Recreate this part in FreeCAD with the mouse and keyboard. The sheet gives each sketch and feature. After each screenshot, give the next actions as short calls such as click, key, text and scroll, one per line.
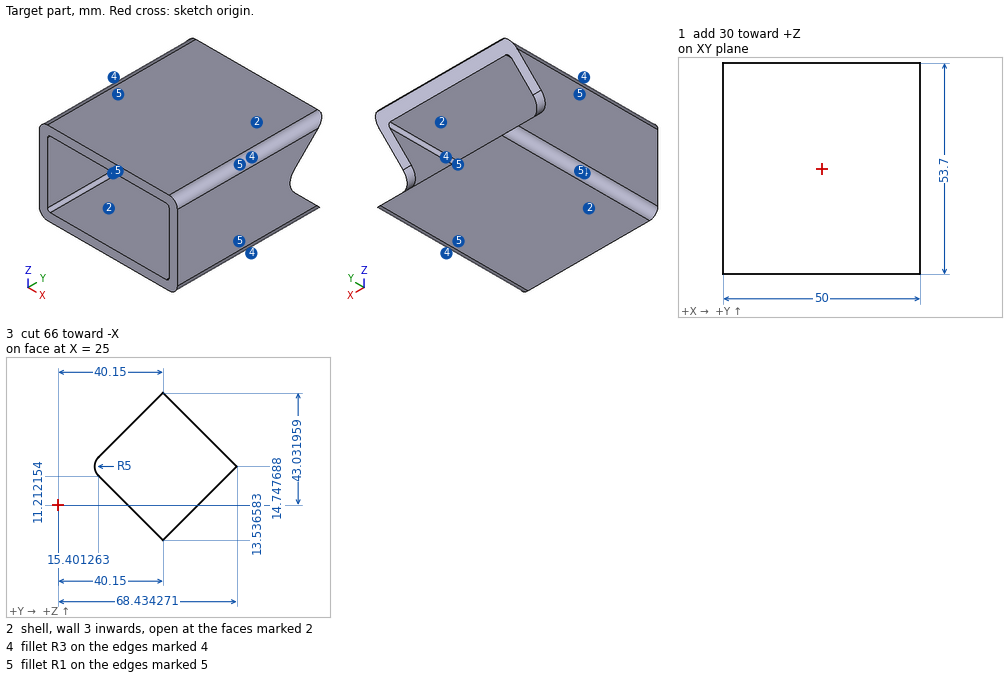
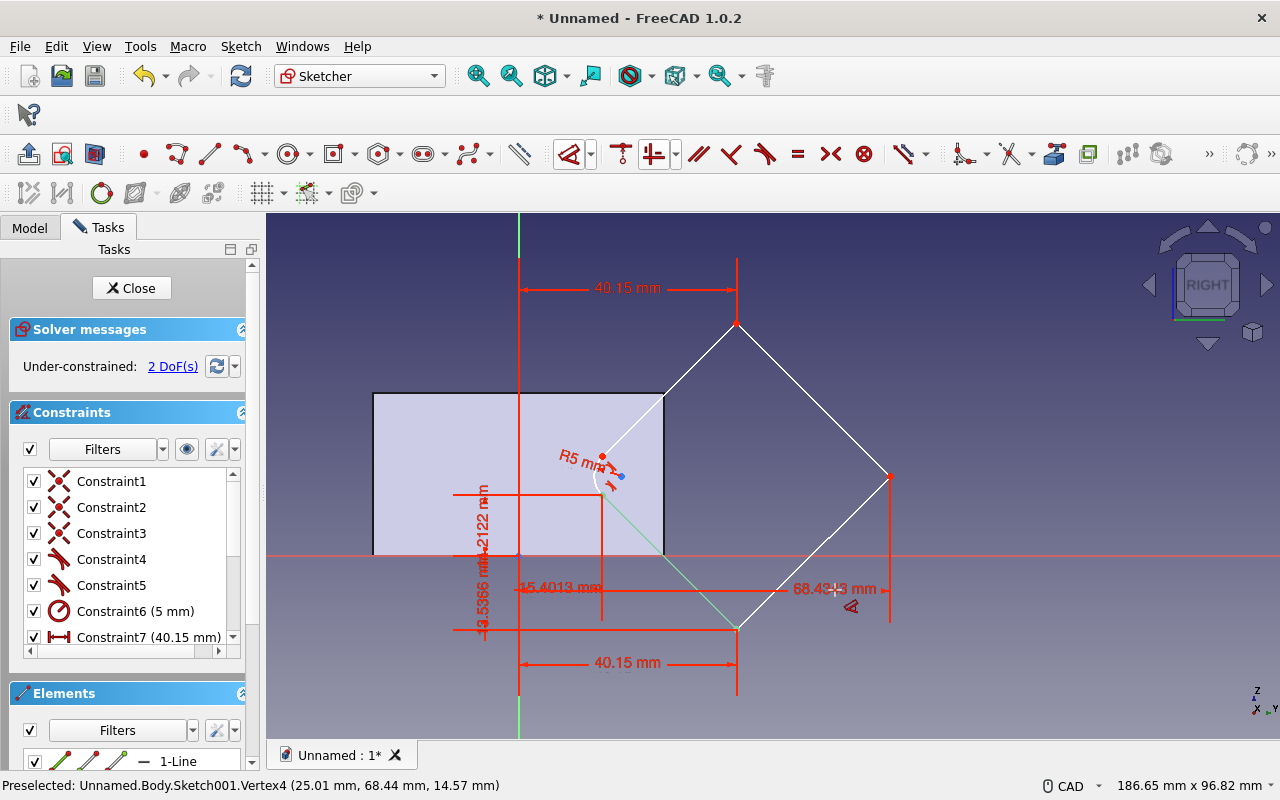
click(890, 477)
click(485, 498)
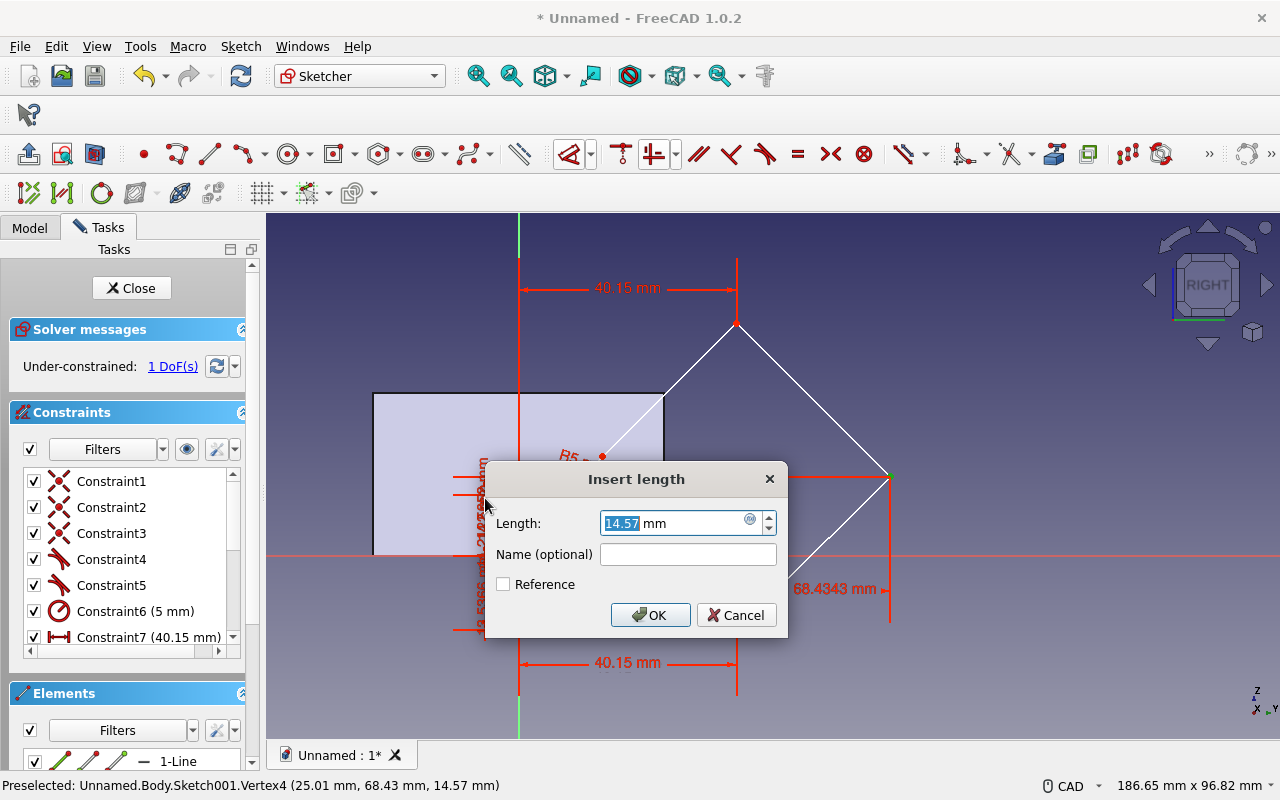
text(14.747688)
key(Return)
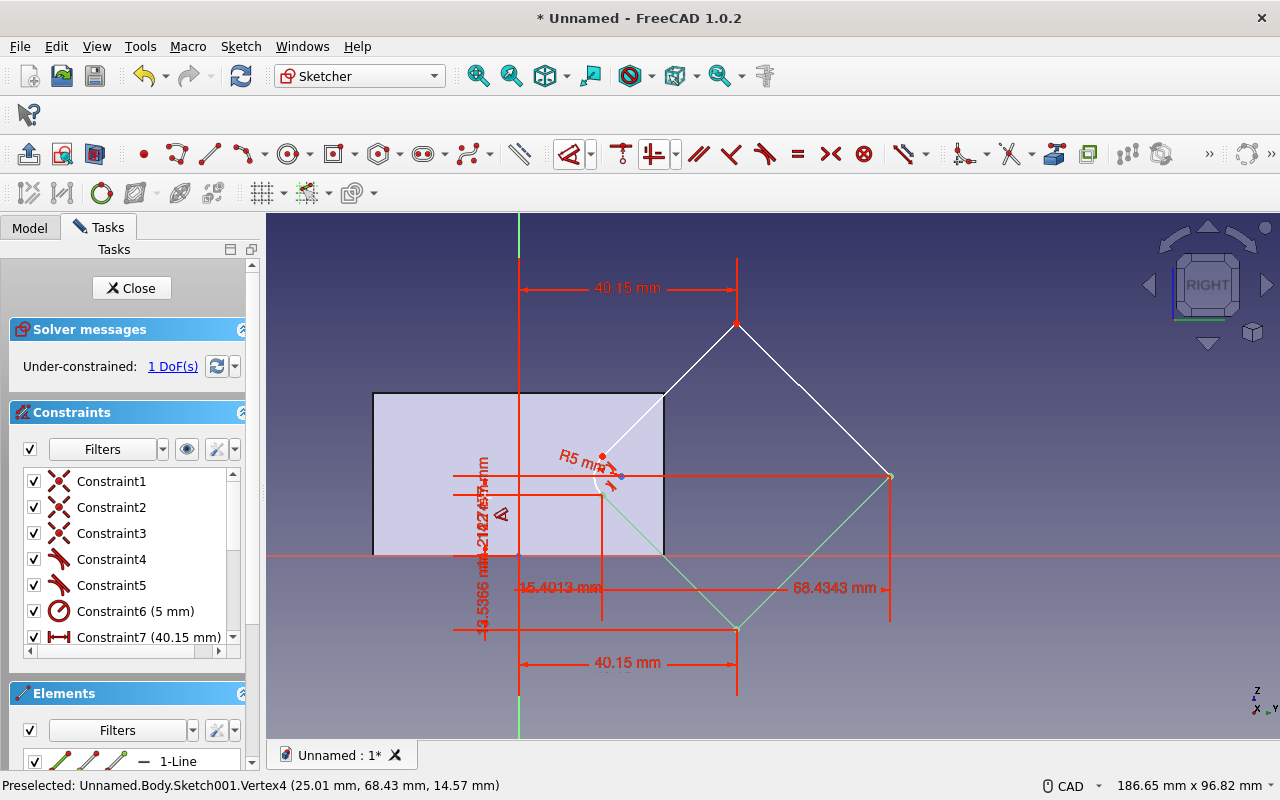
click(737, 323)
click(485, 440)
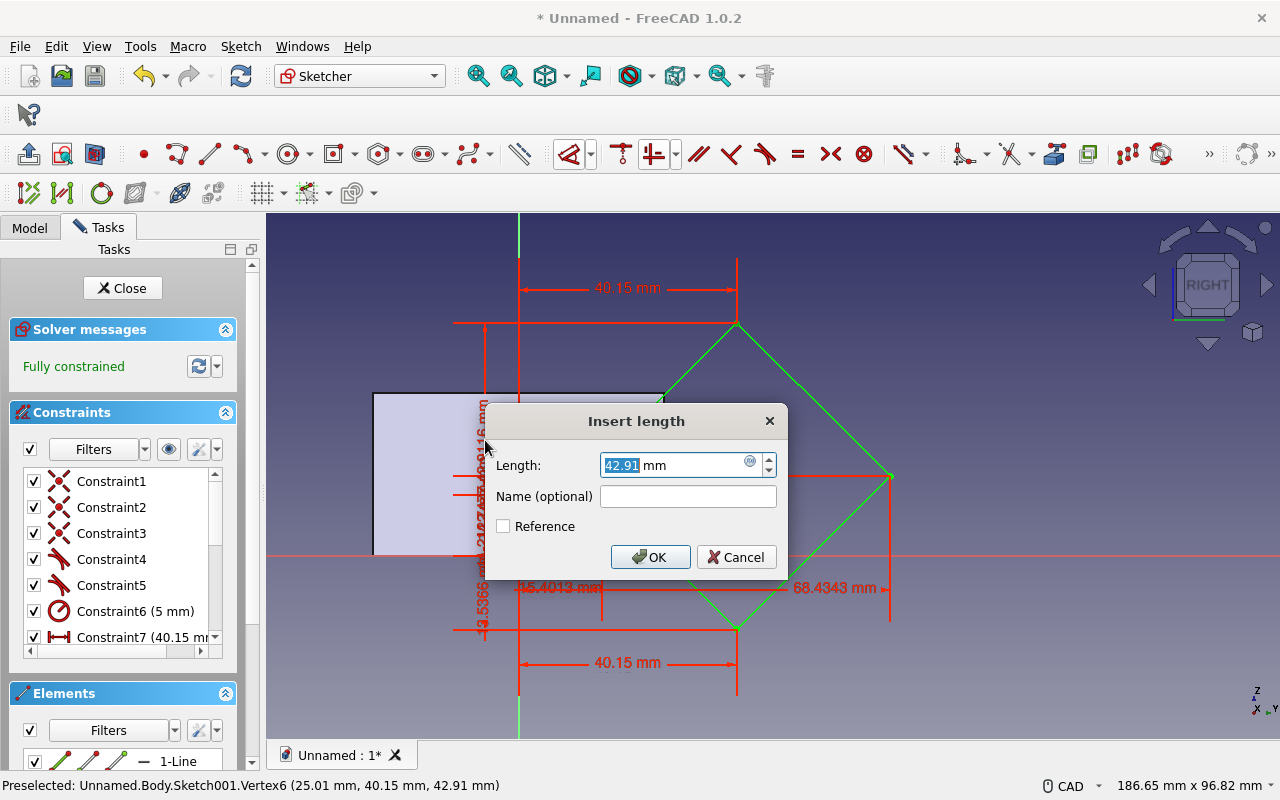
text(43.031959)
key(Return)
key(Escape)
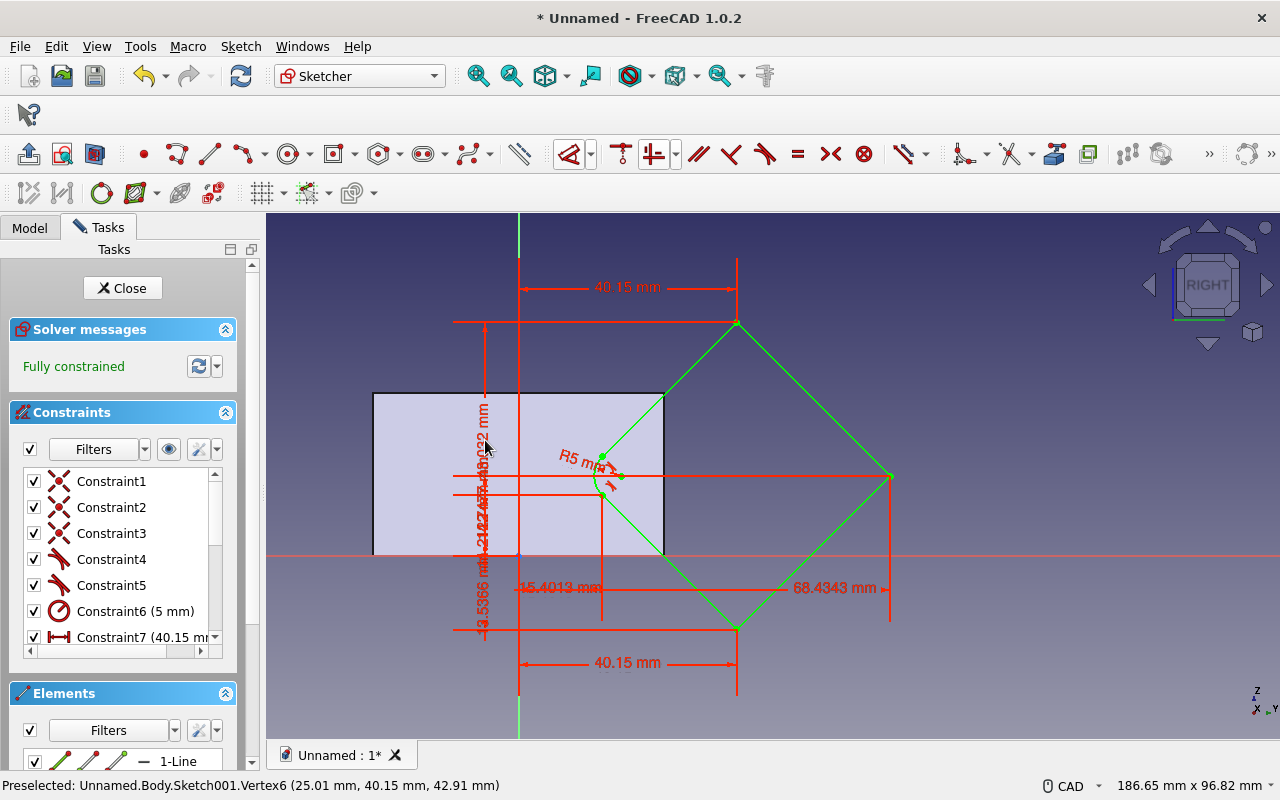
click(123, 288)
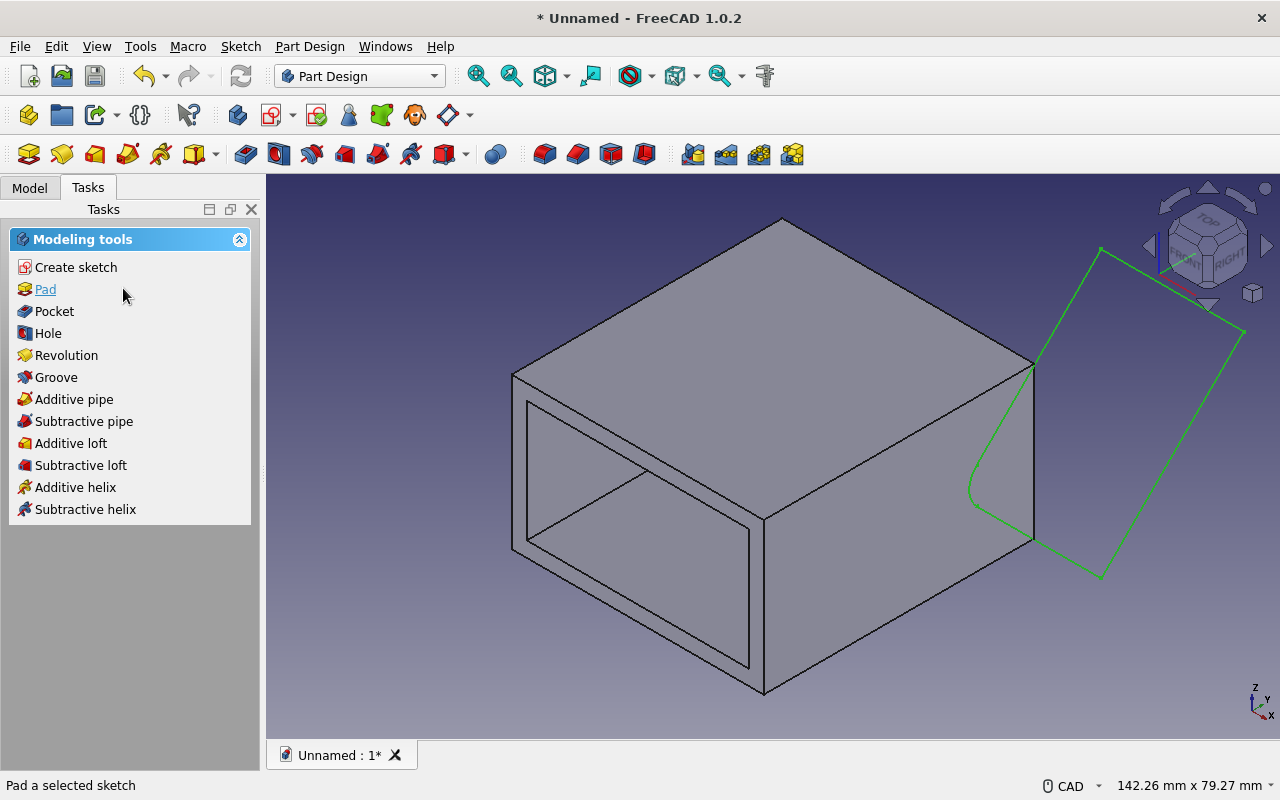
click(246, 154)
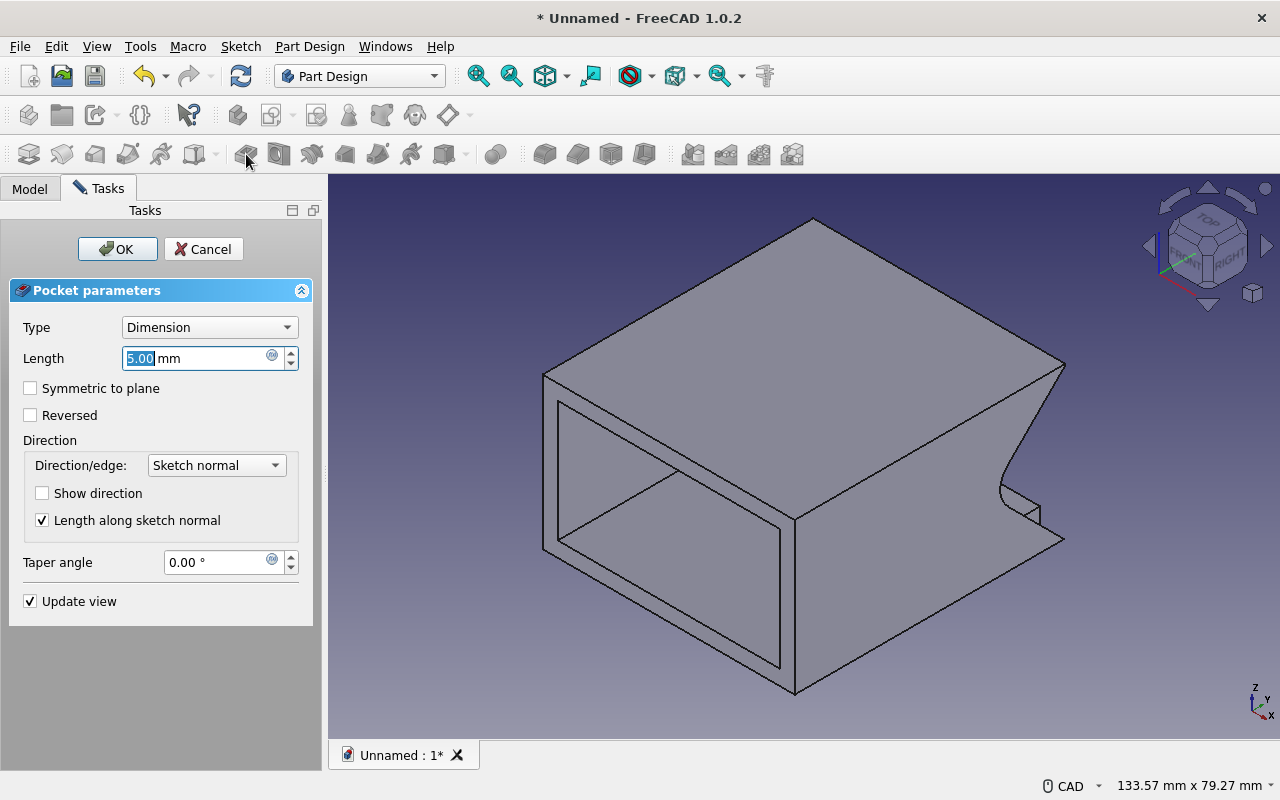
text(66)
key(Tab)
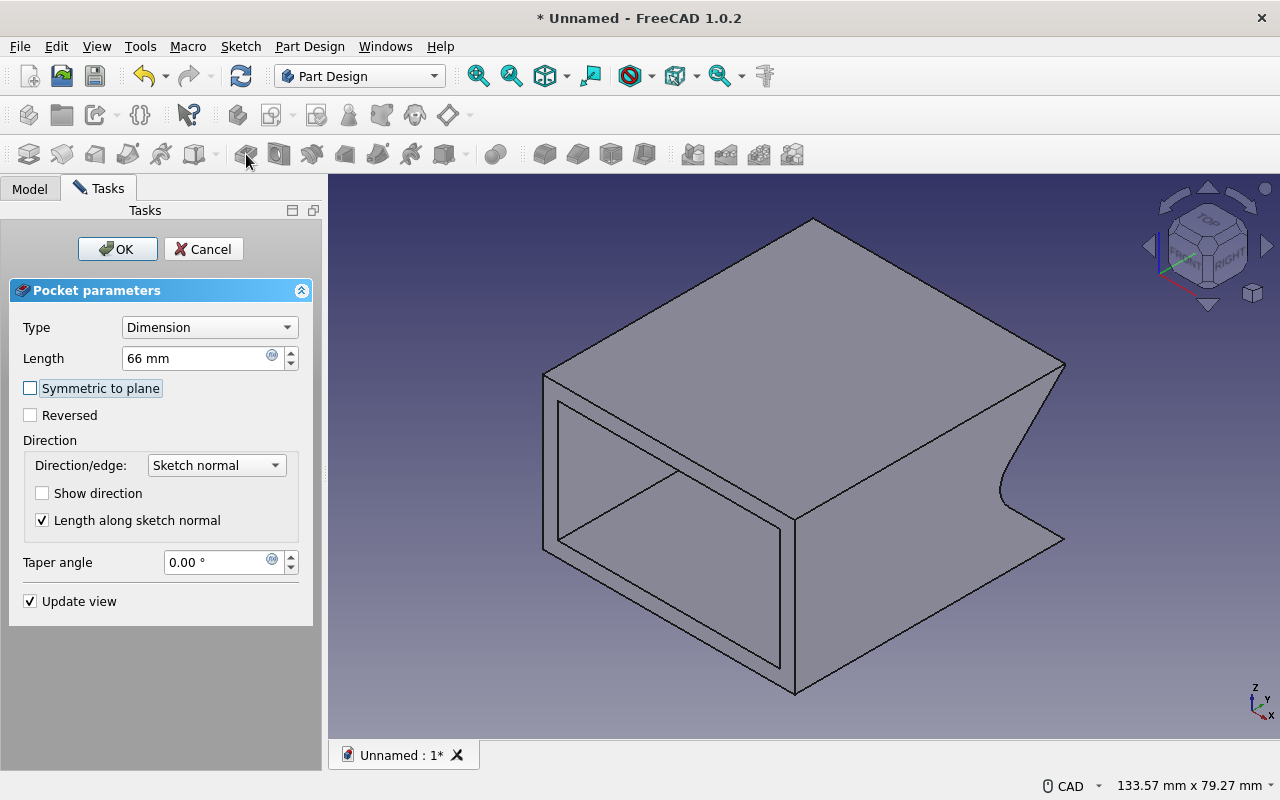
click(118, 249)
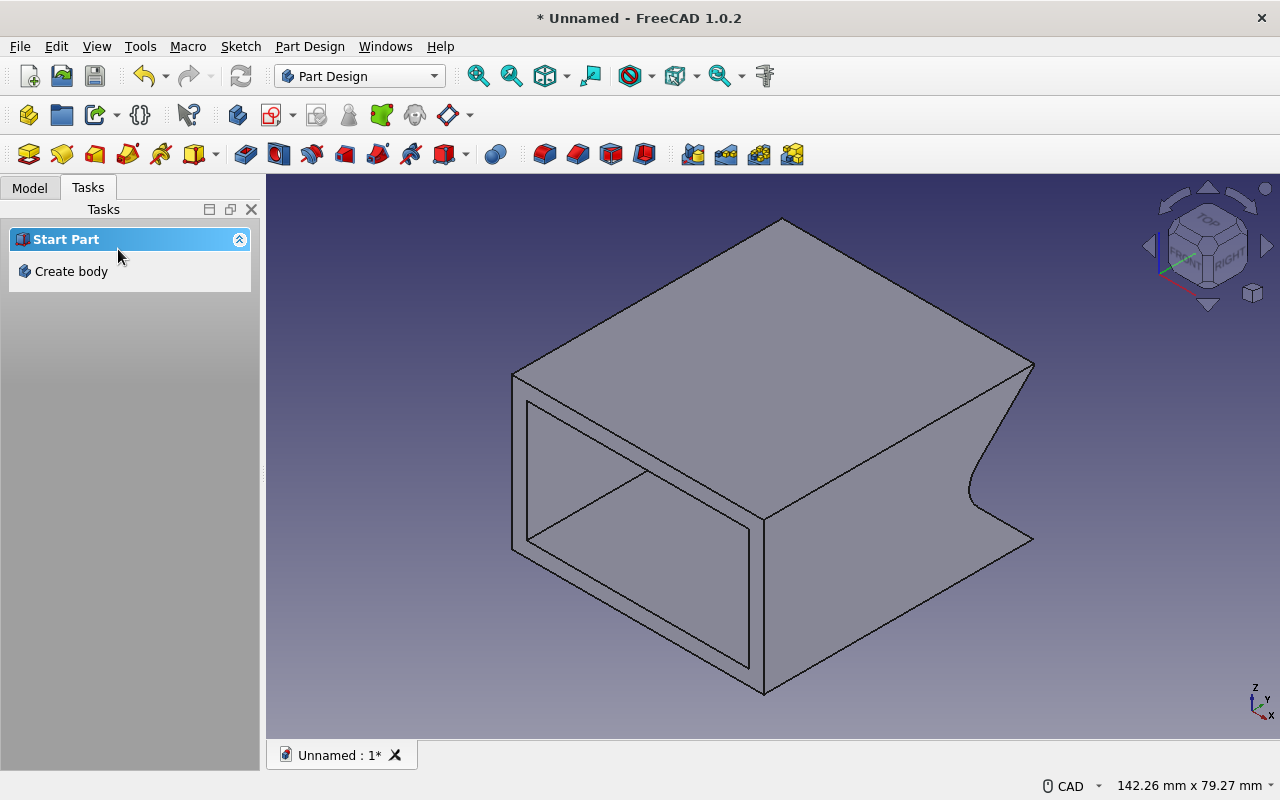
click(899, 441)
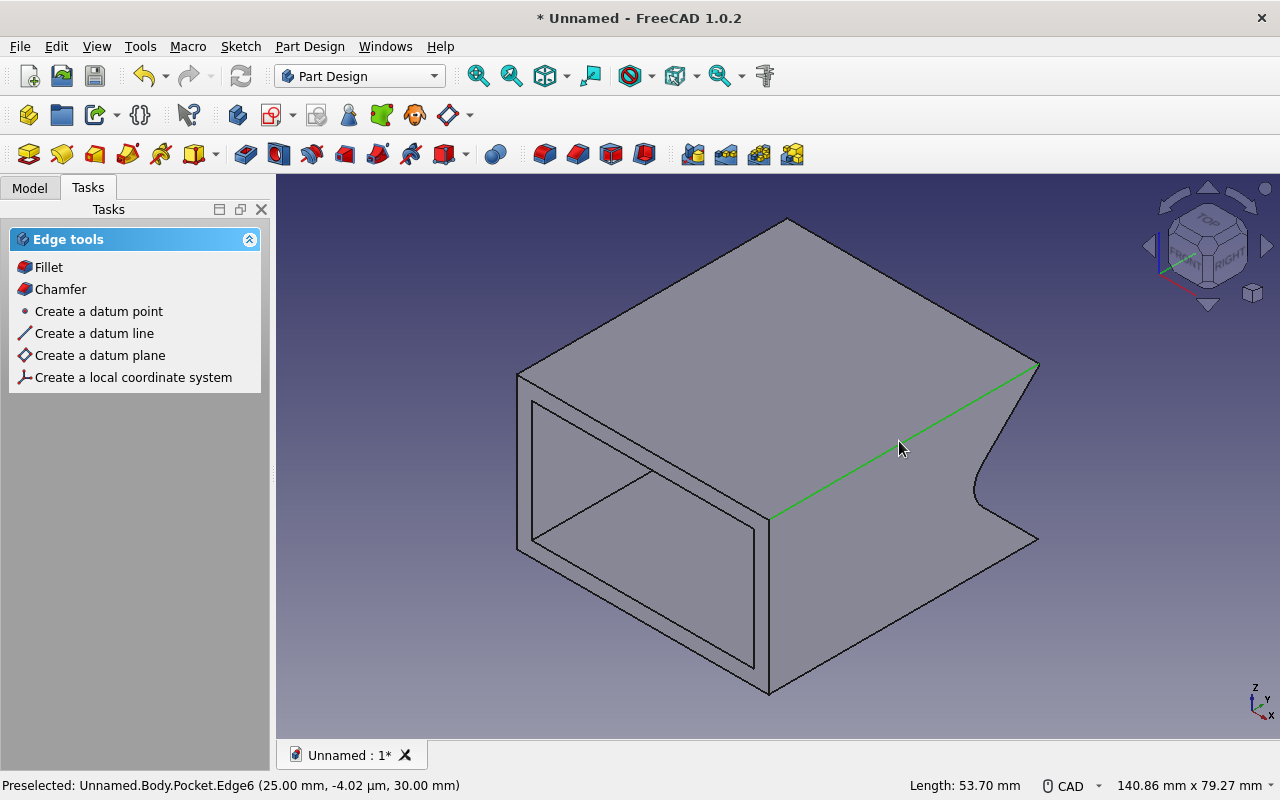
key(2)